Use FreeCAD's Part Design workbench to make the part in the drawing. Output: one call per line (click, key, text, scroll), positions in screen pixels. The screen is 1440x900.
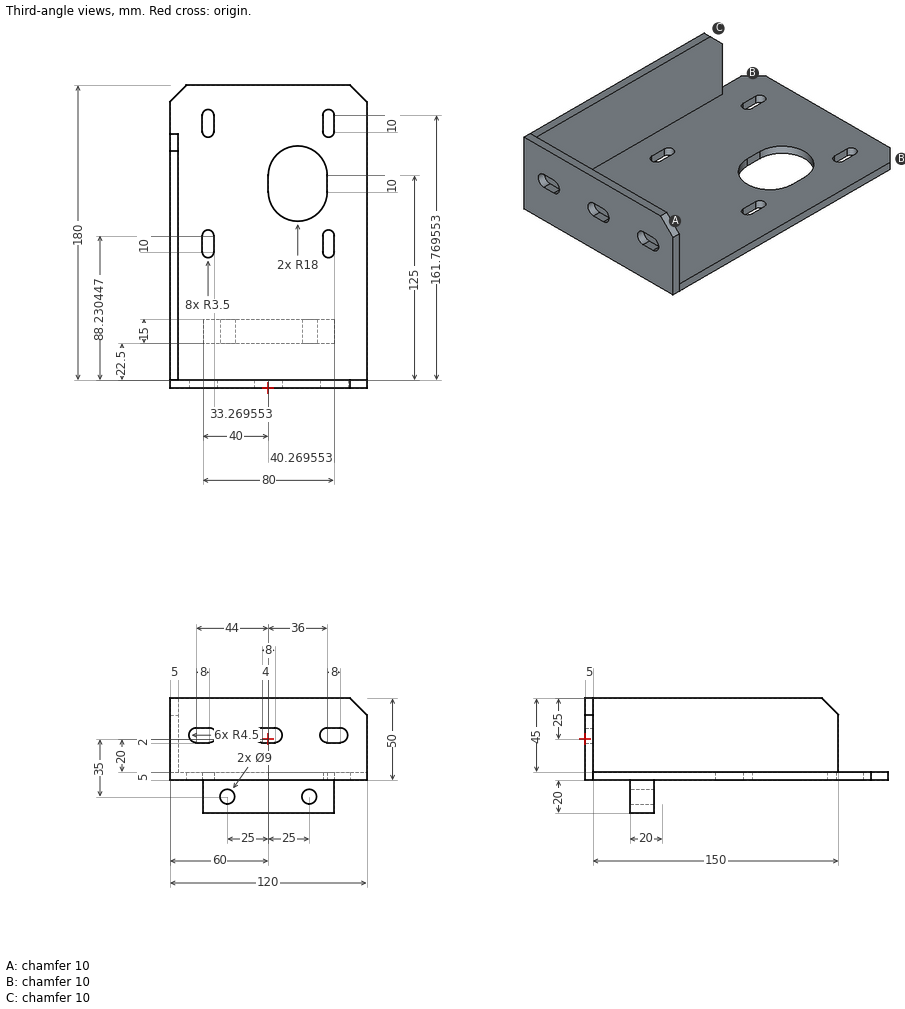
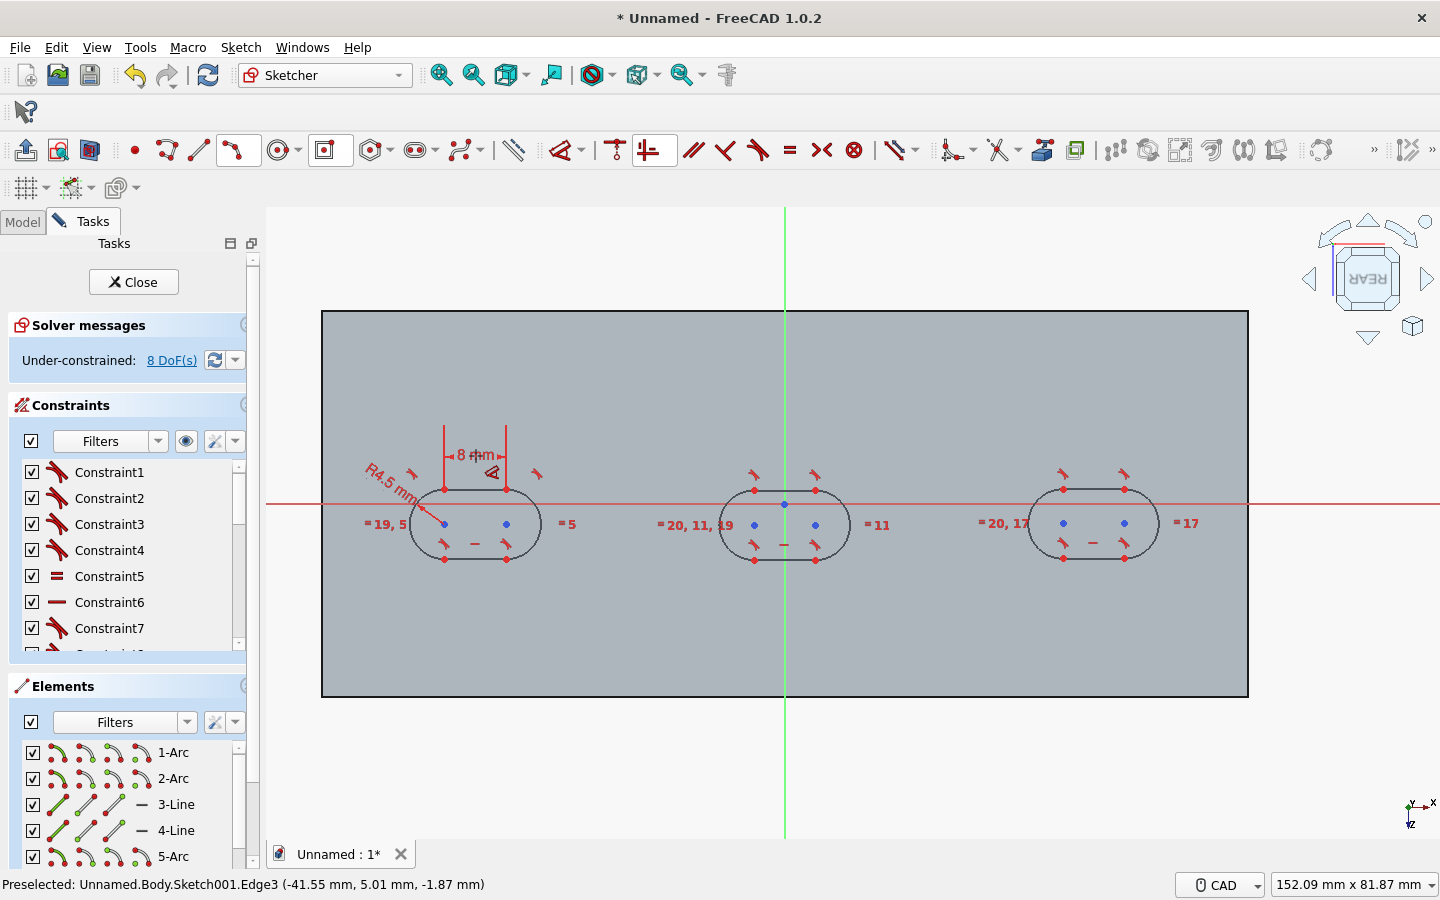
click(773, 491)
click(771, 457)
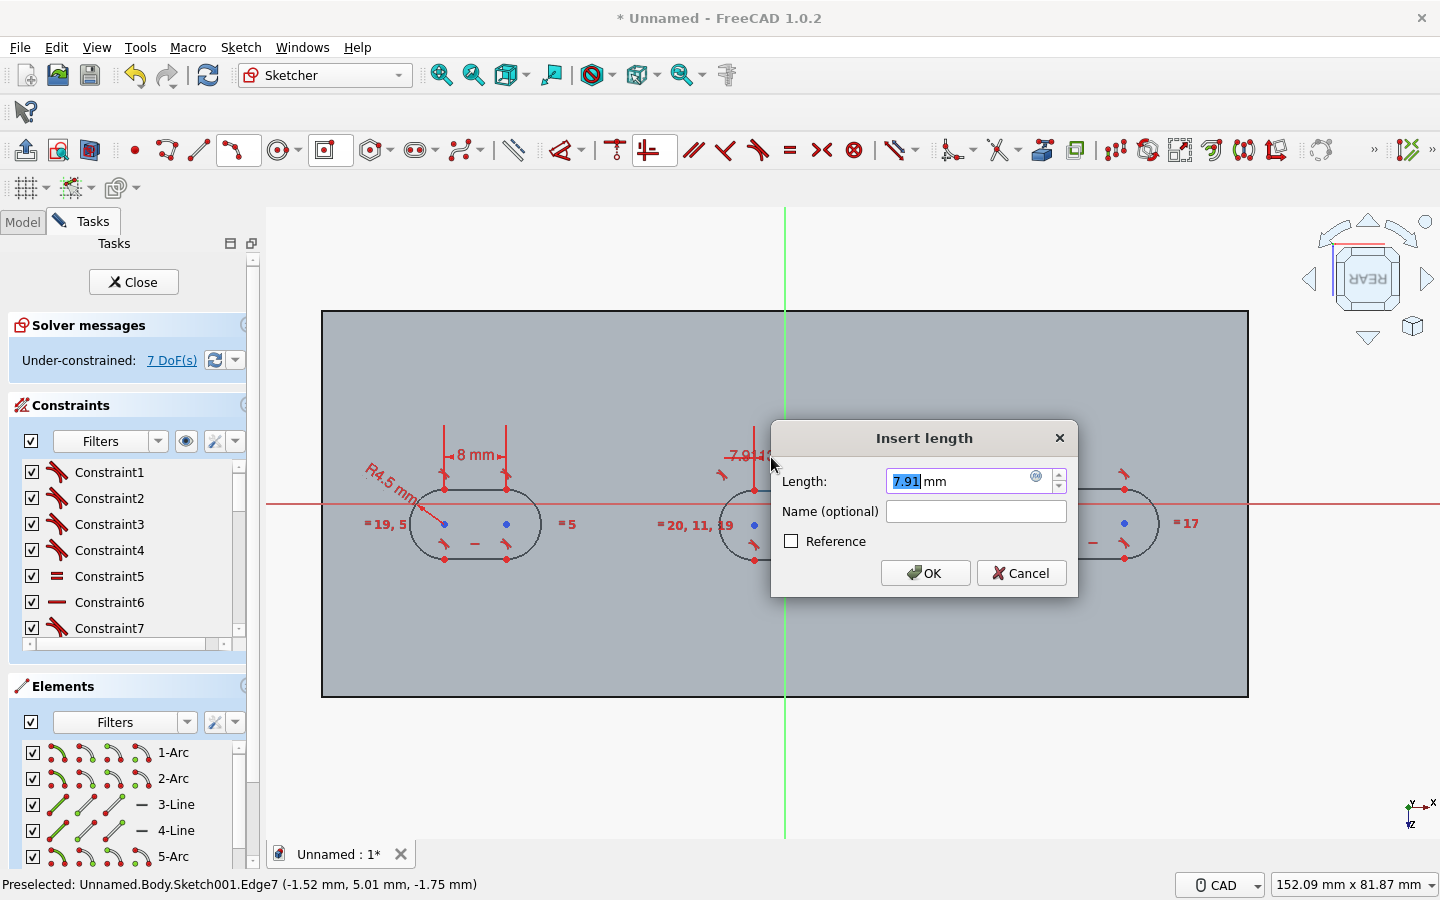
text(8)
key(Return)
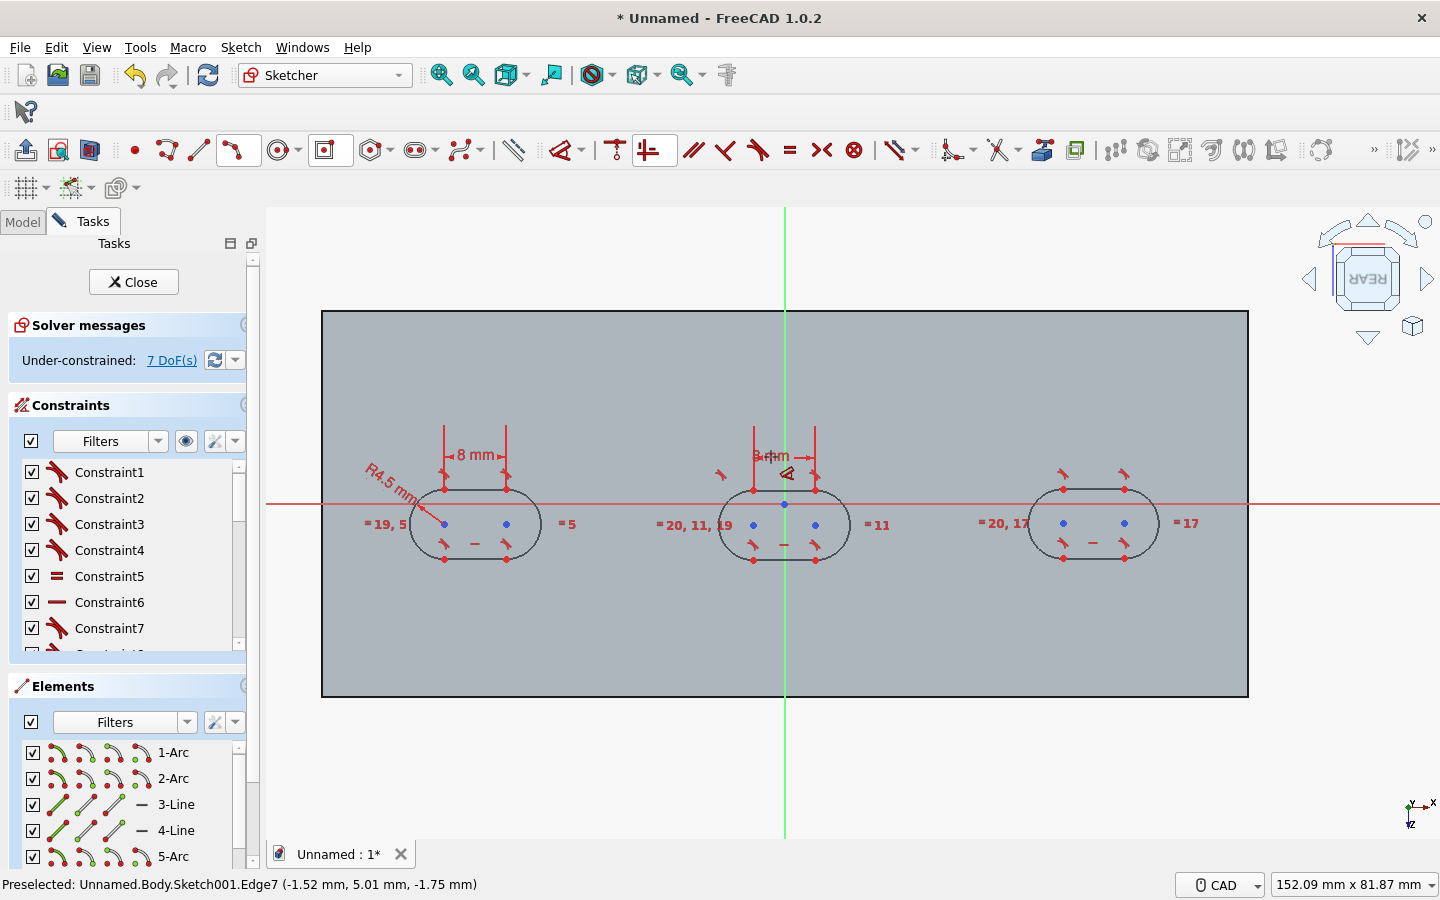
click(1081, 489)
click(1094, 455)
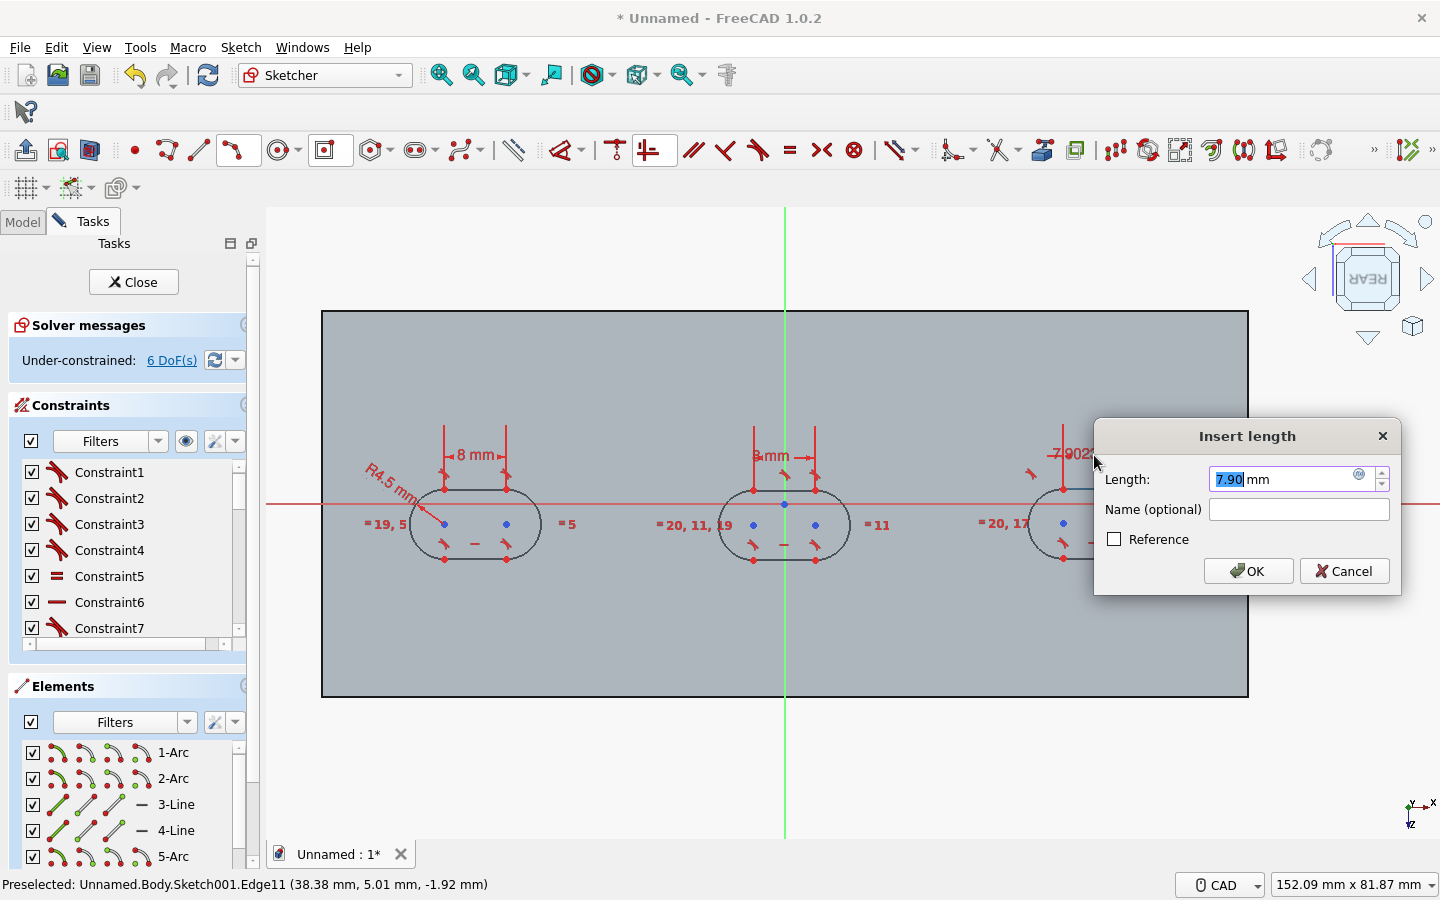
text(8)
key(Return)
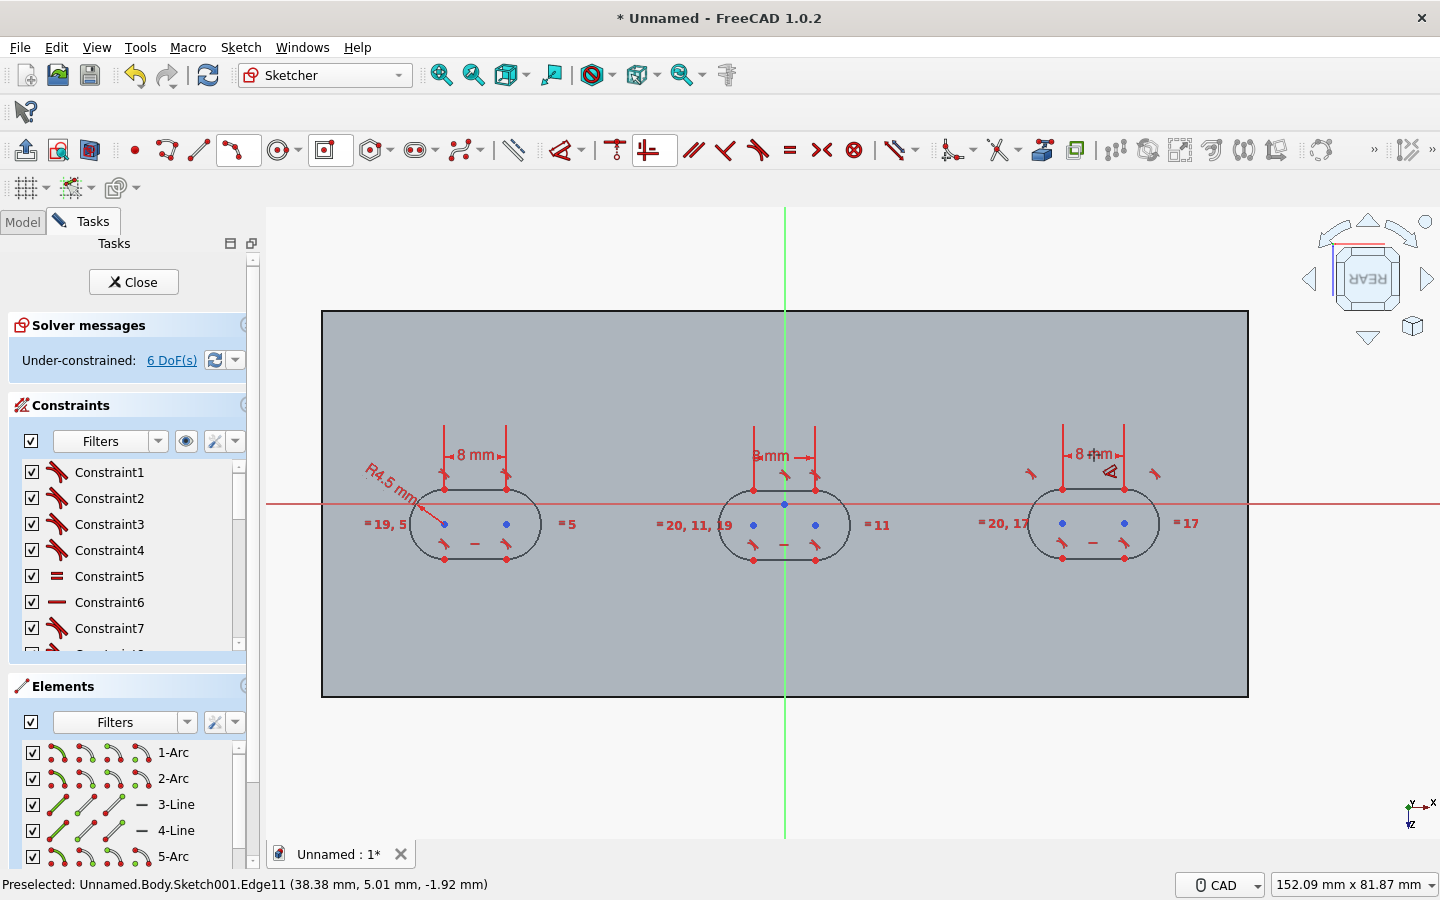
scroll(445, 490, up, 5)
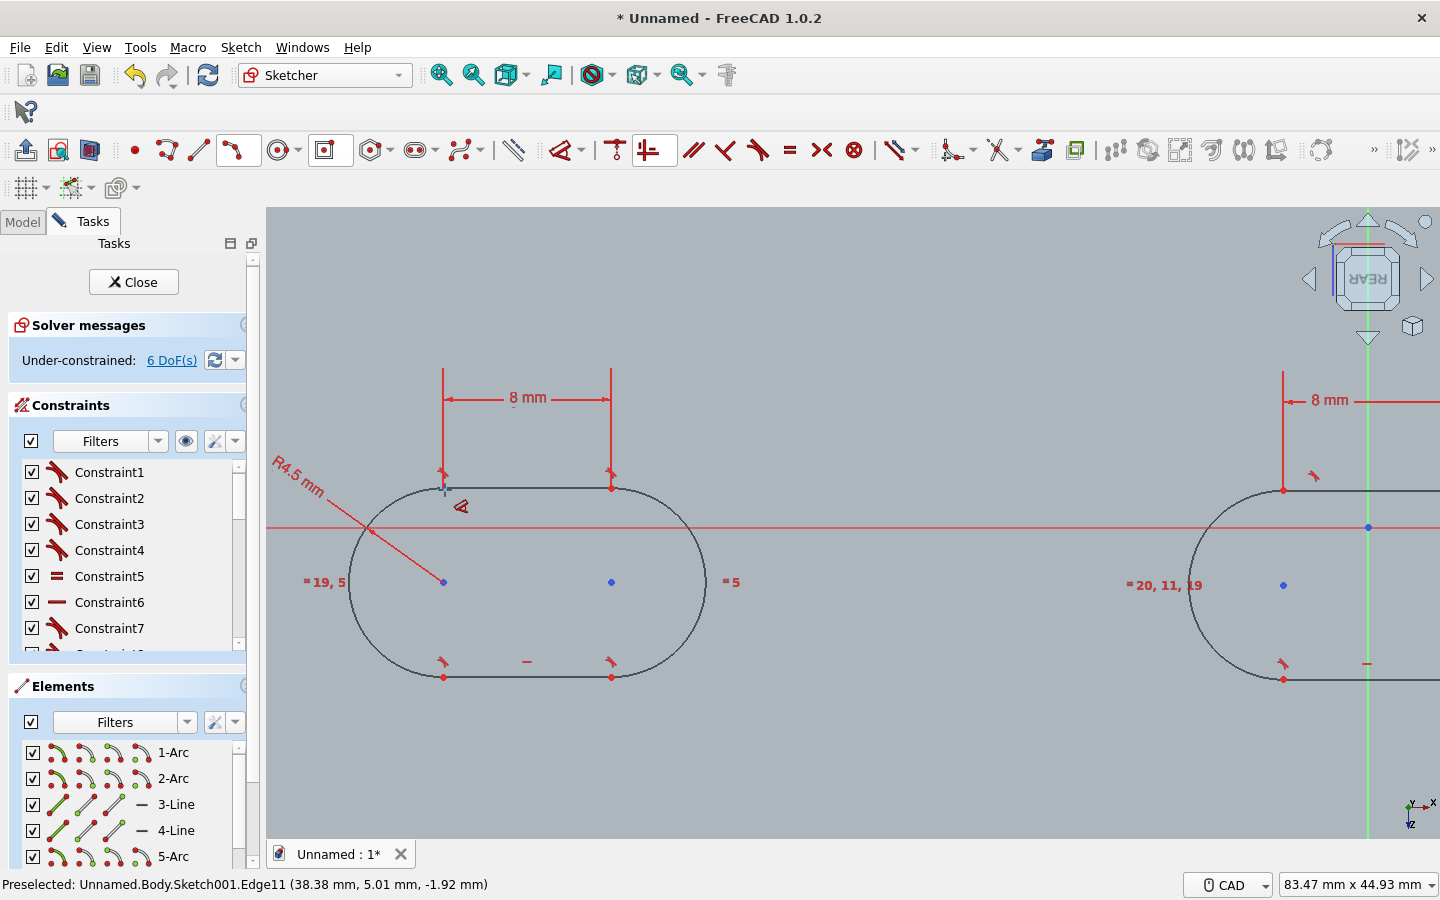
click(443, 488)
click(361, 508)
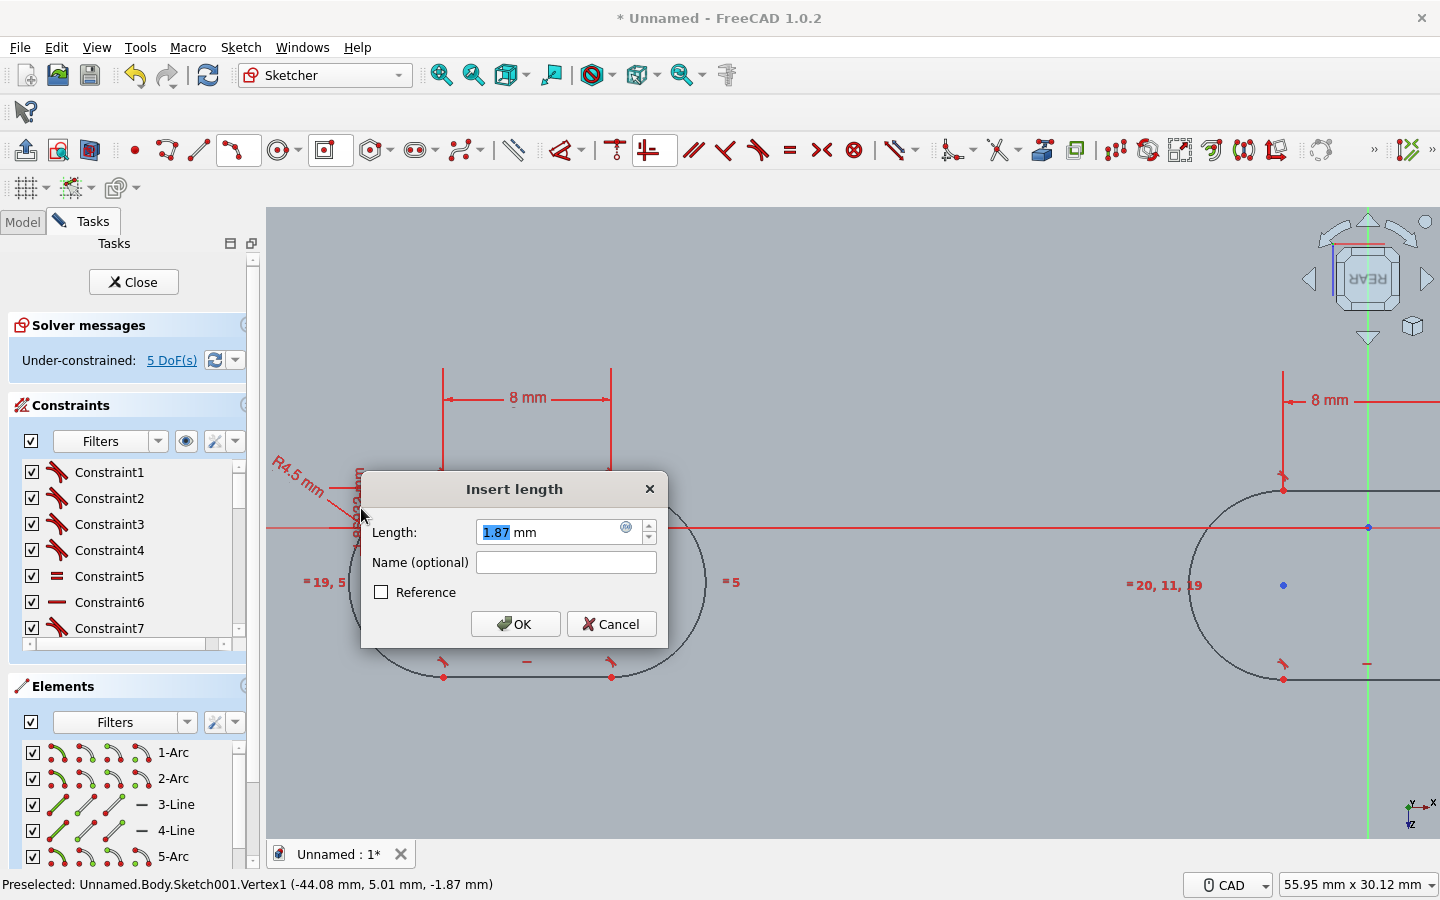
text(2)
key(Return)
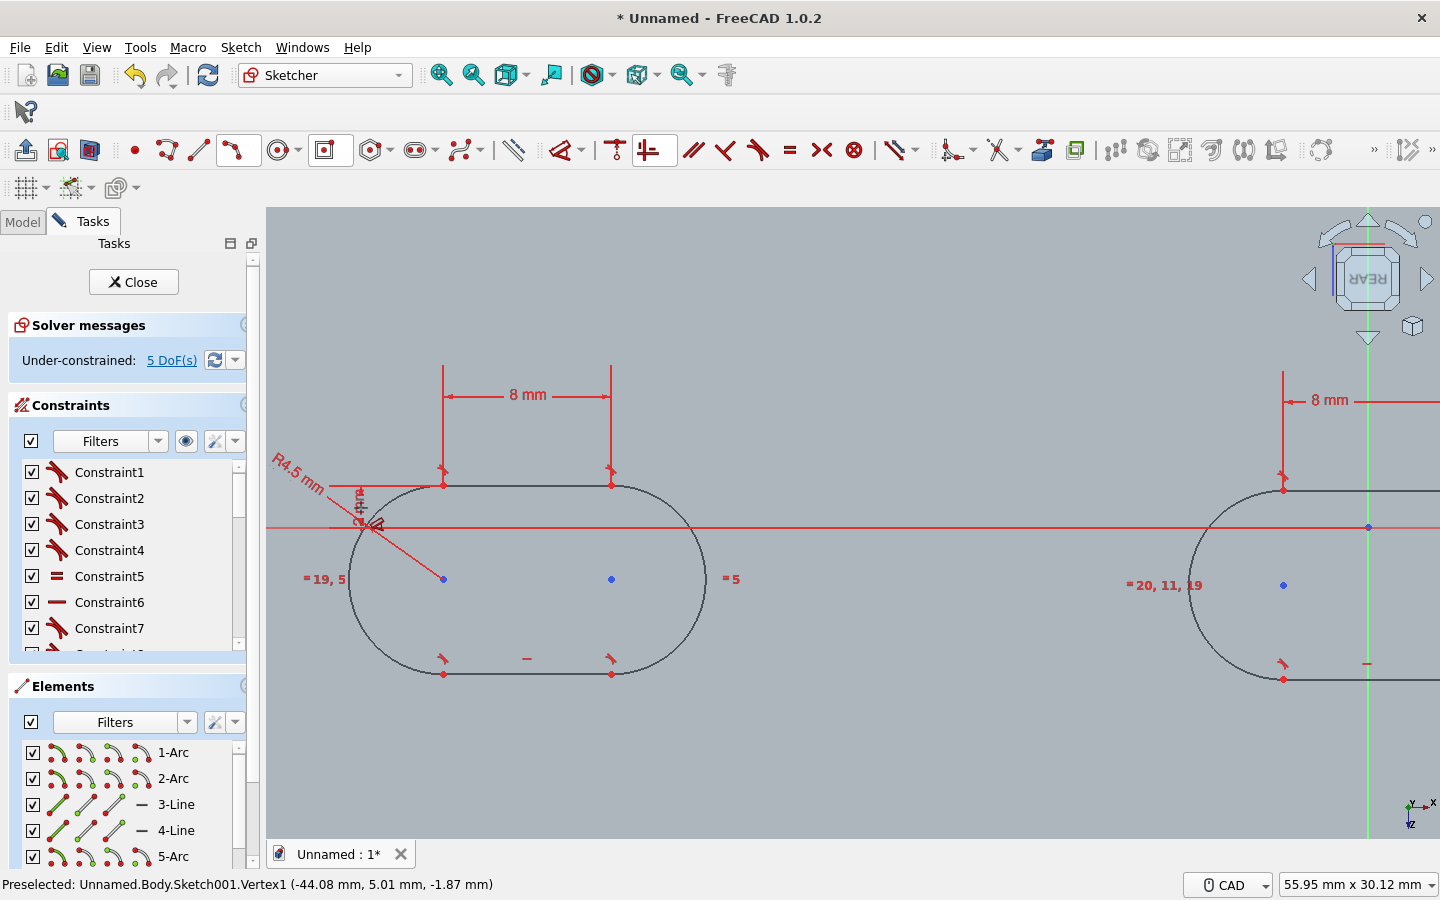
scroll(445, 490, down, 5)